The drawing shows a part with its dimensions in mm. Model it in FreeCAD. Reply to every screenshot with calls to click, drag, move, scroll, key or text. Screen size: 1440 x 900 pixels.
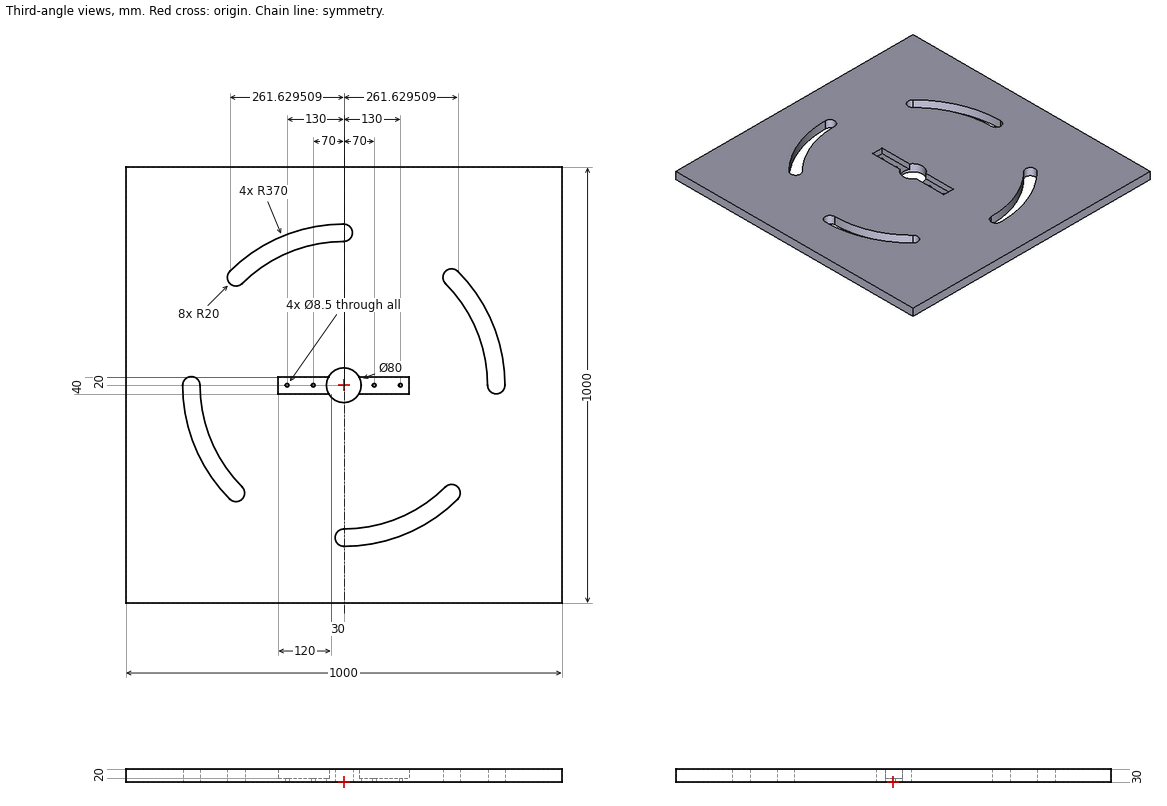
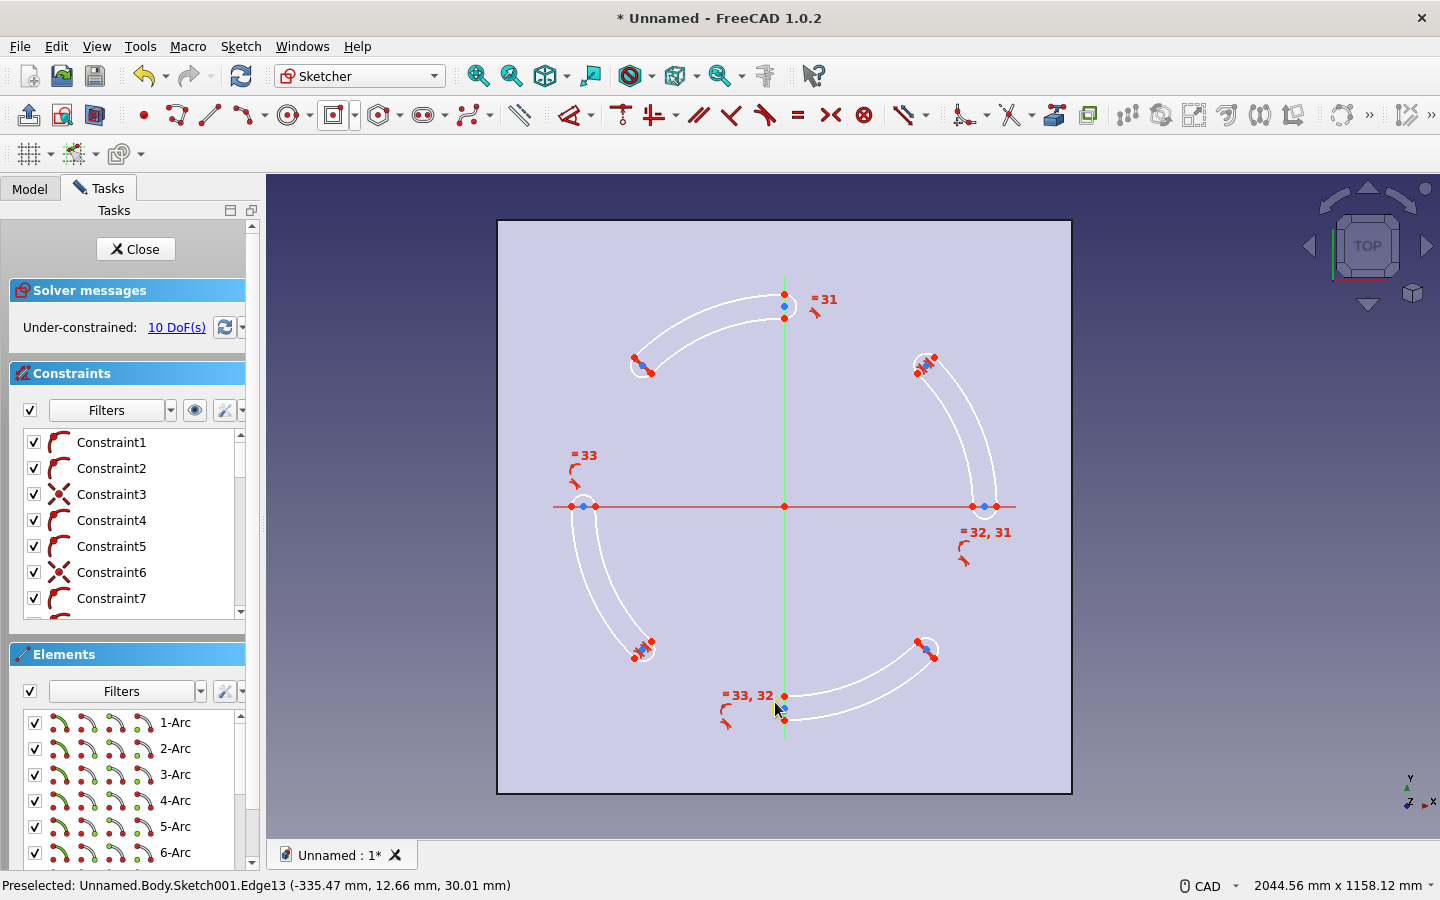
click(735, 301)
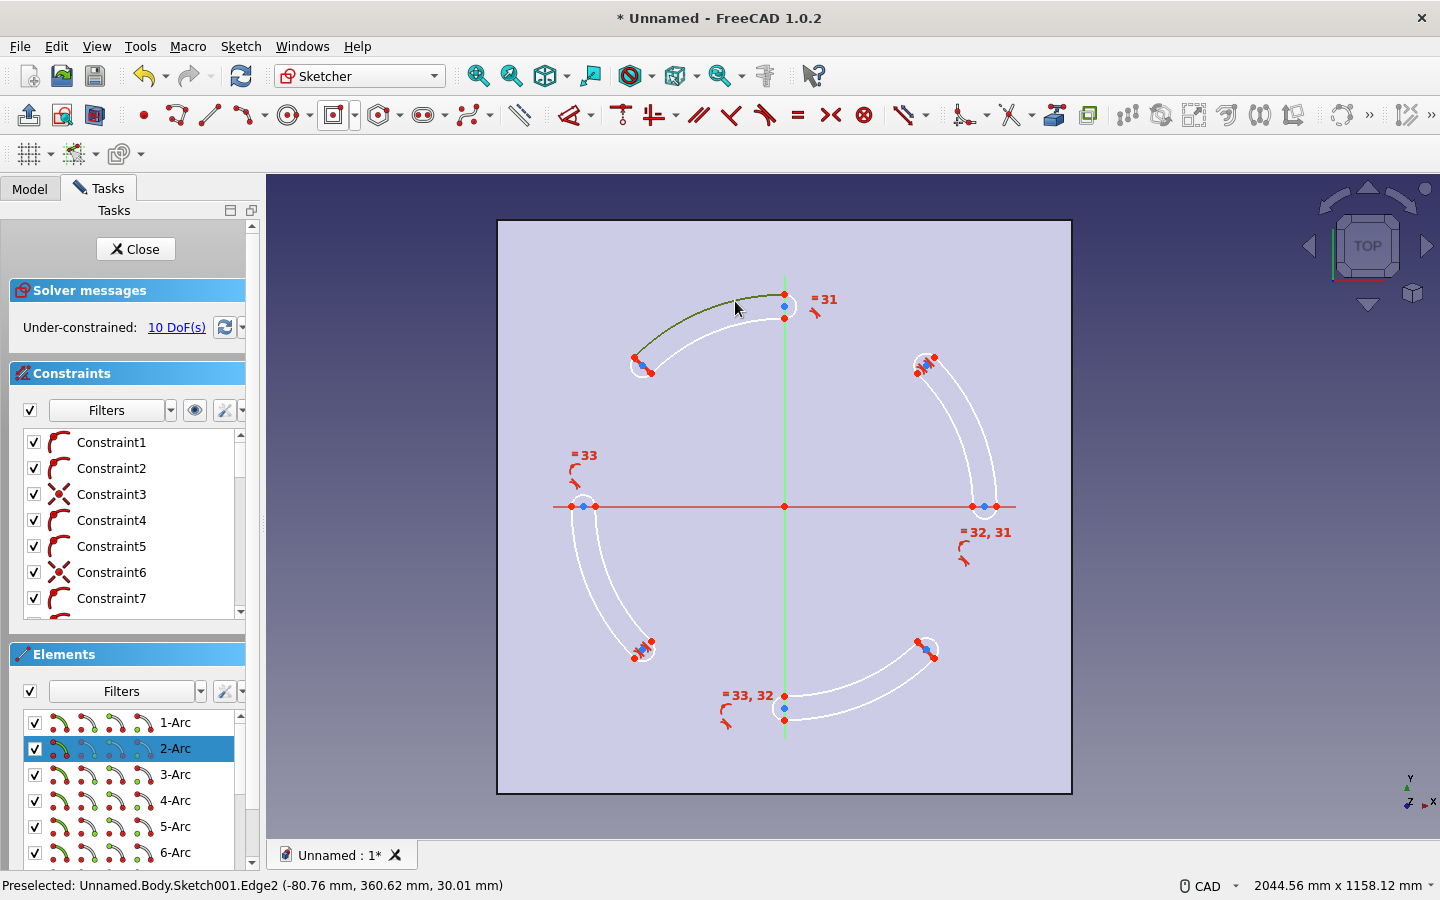
click(991, 458)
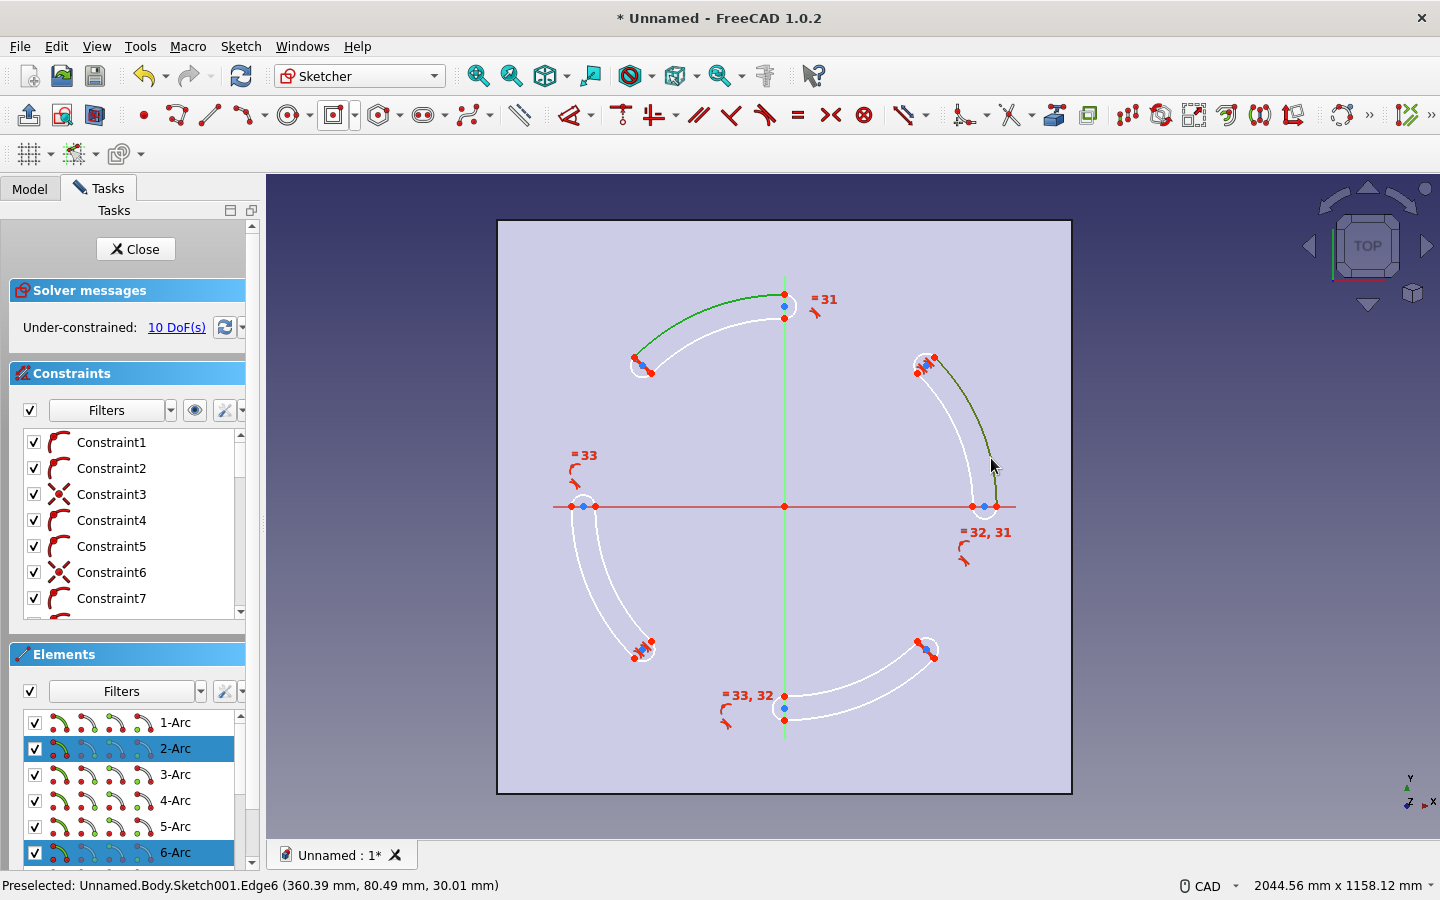
click(834, 714)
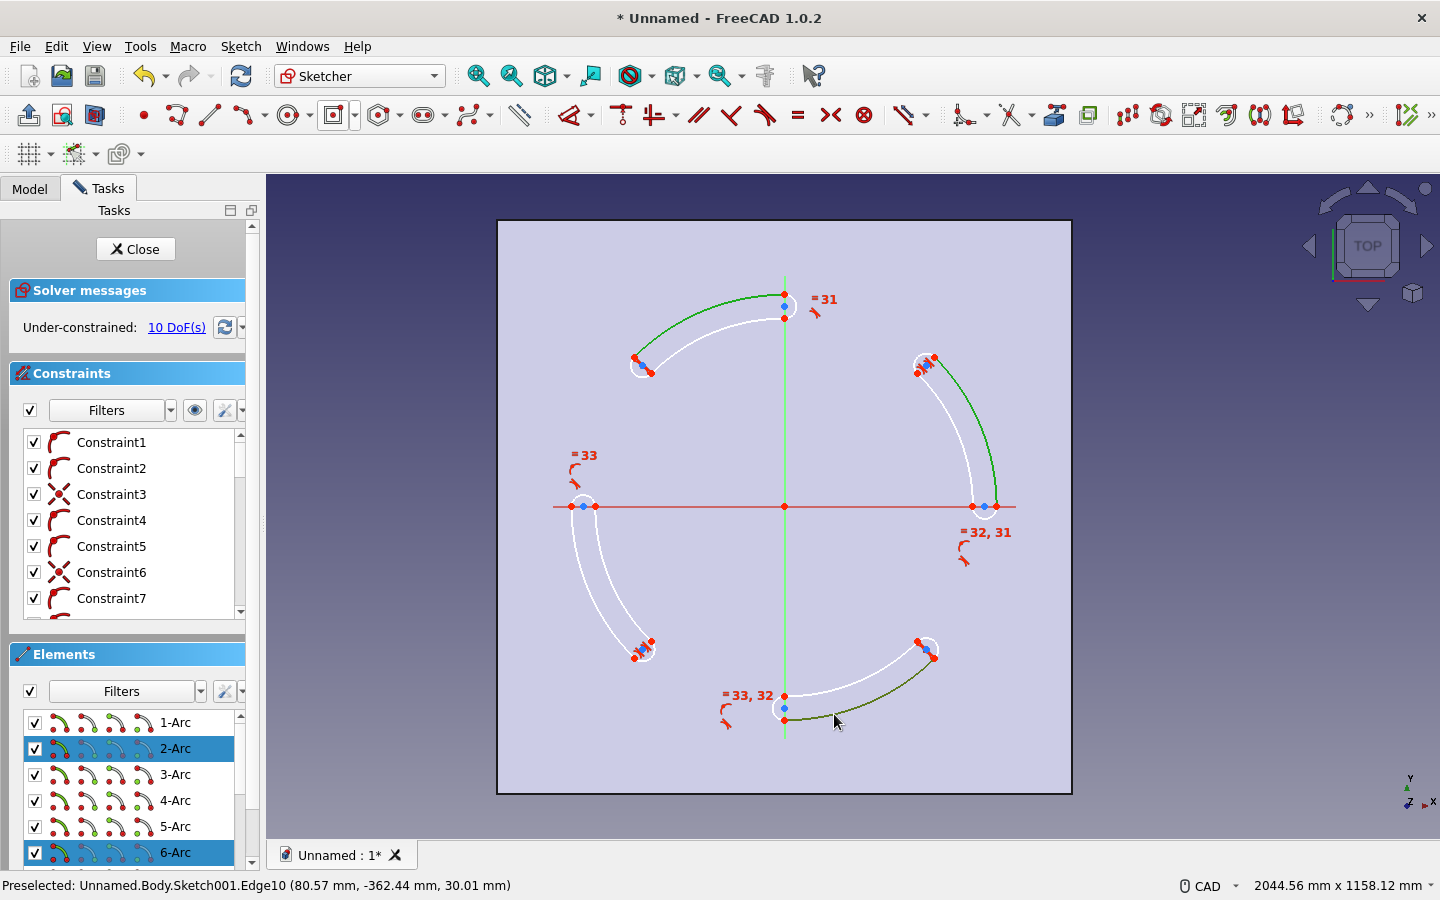
click(578, 557)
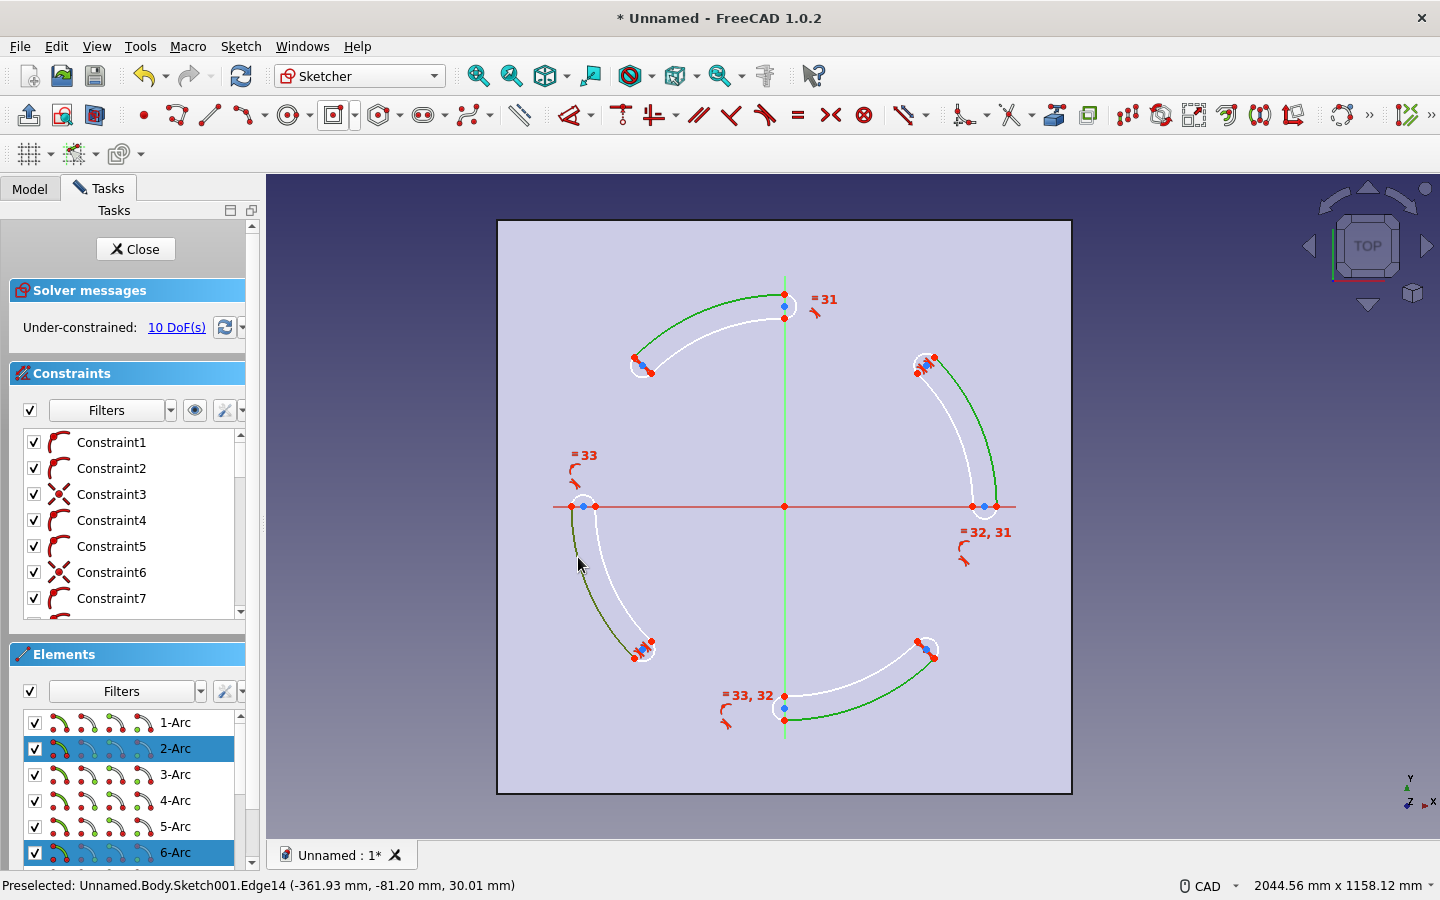
click(798, 116)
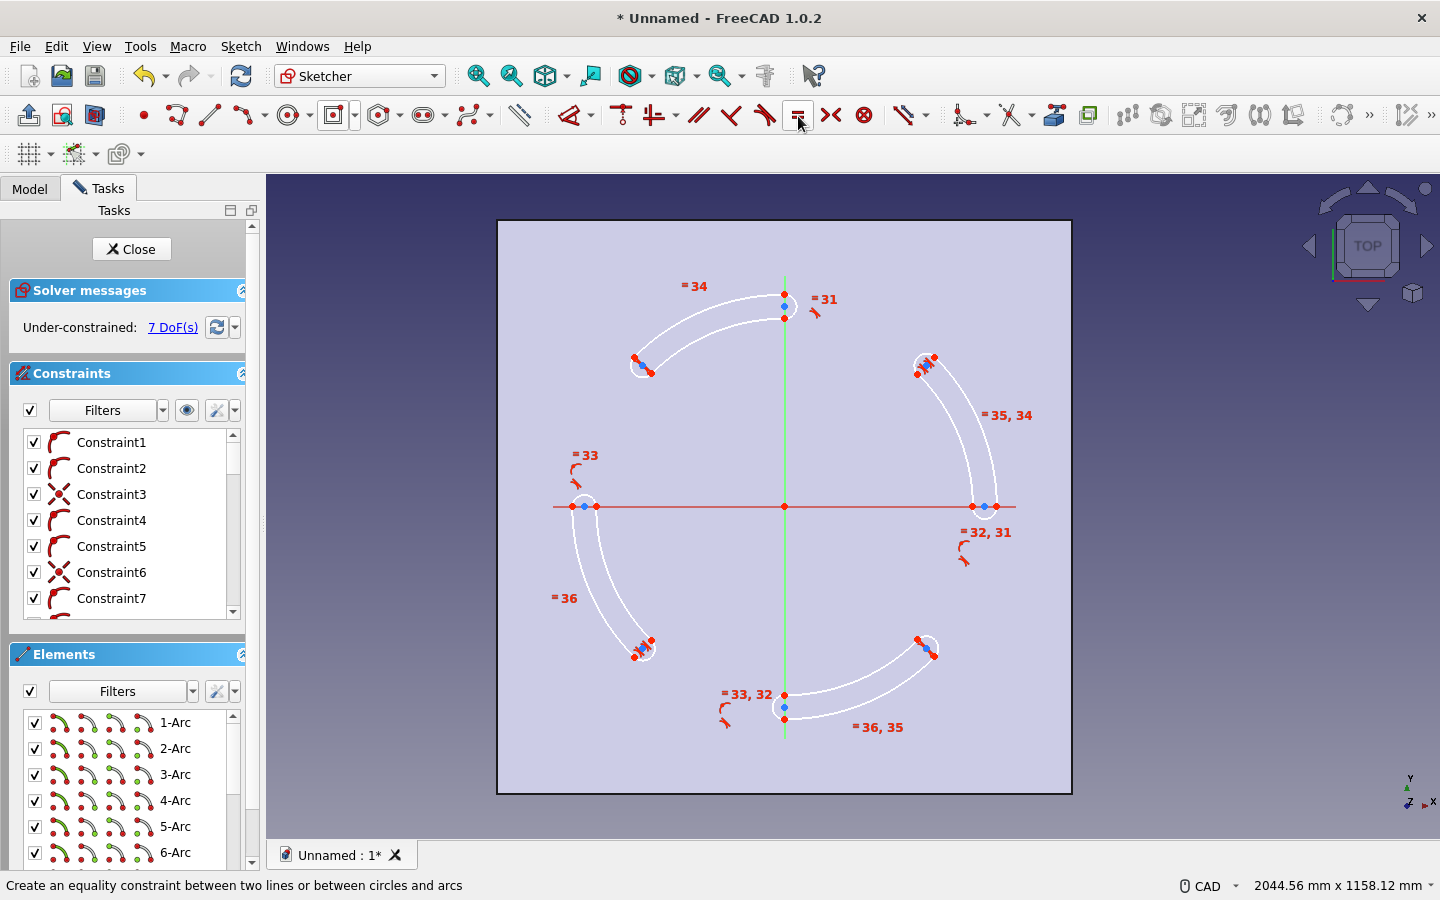
click(785, 307)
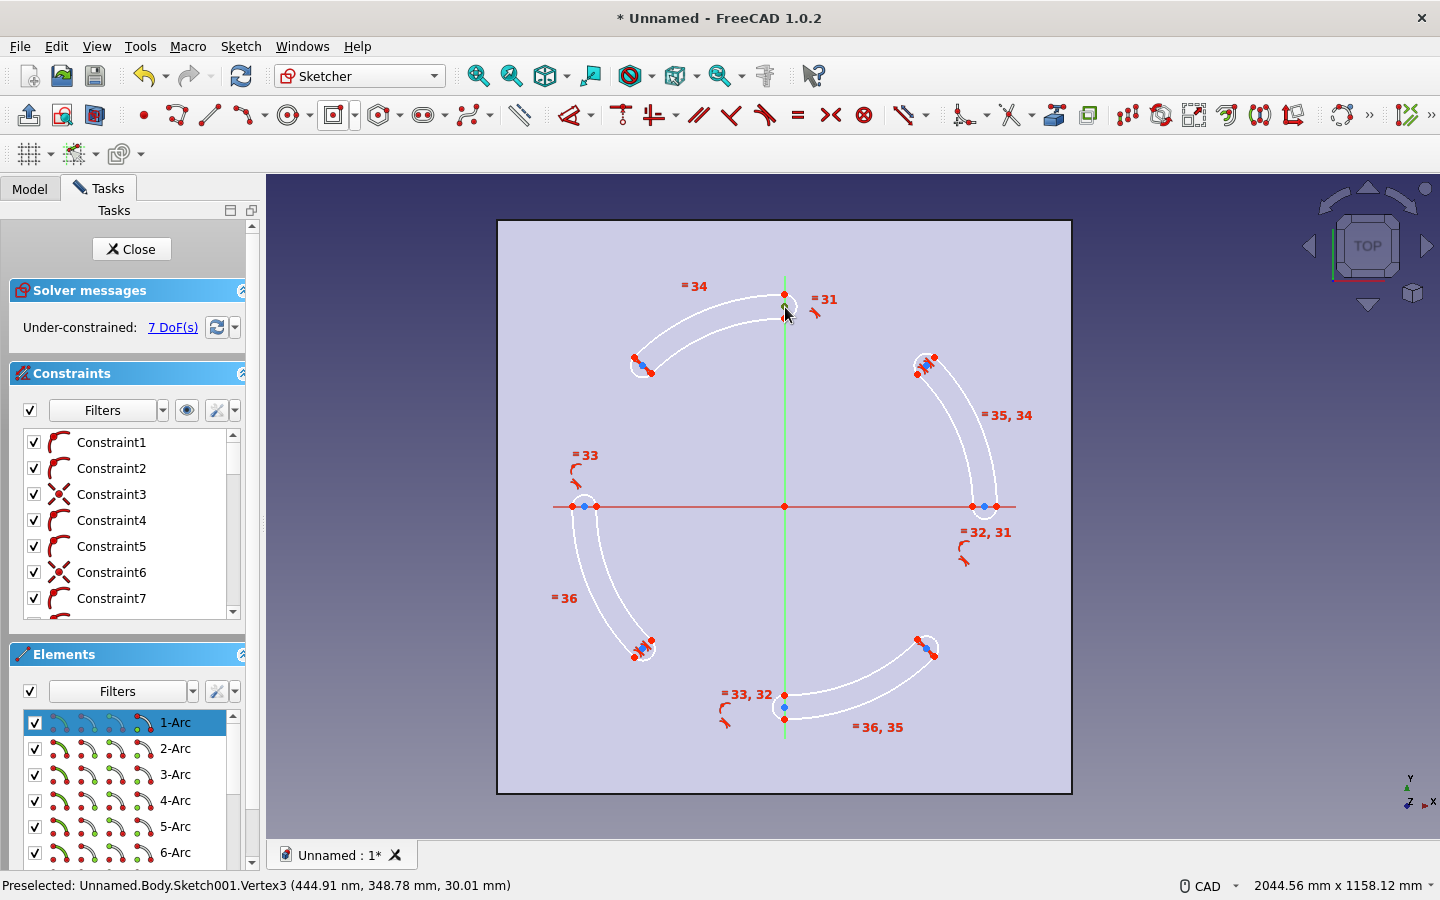
click(785, 637)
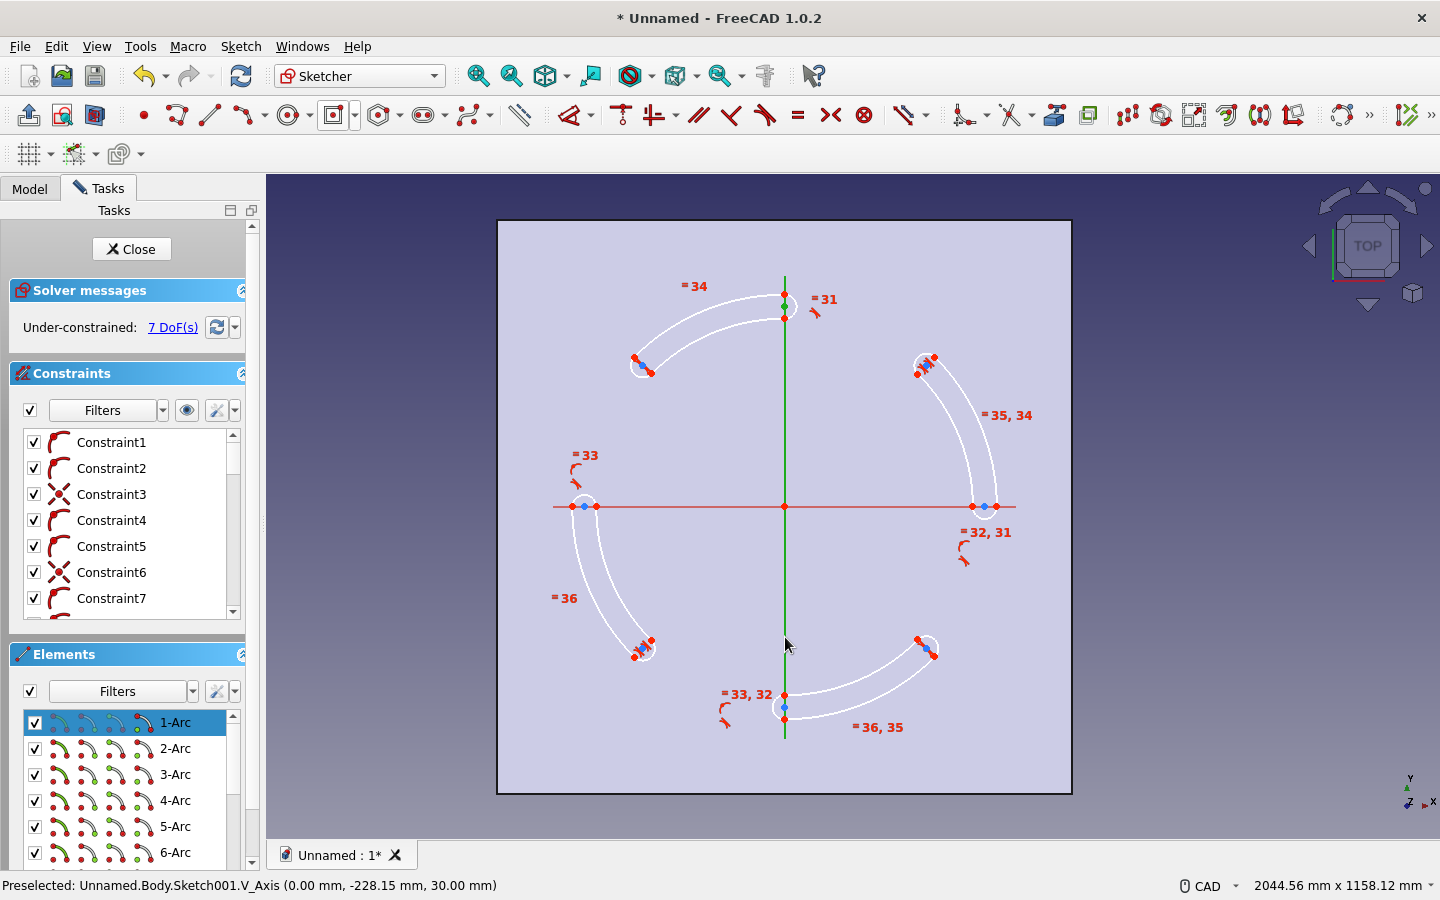
click(621, 116)